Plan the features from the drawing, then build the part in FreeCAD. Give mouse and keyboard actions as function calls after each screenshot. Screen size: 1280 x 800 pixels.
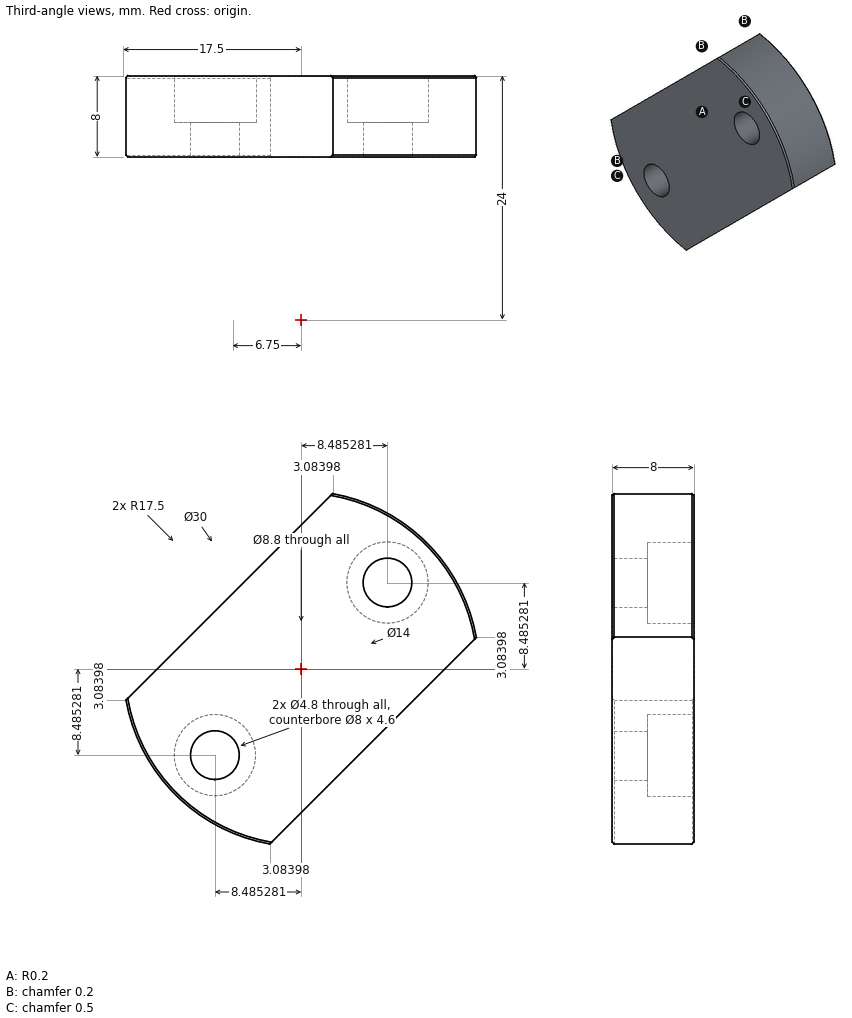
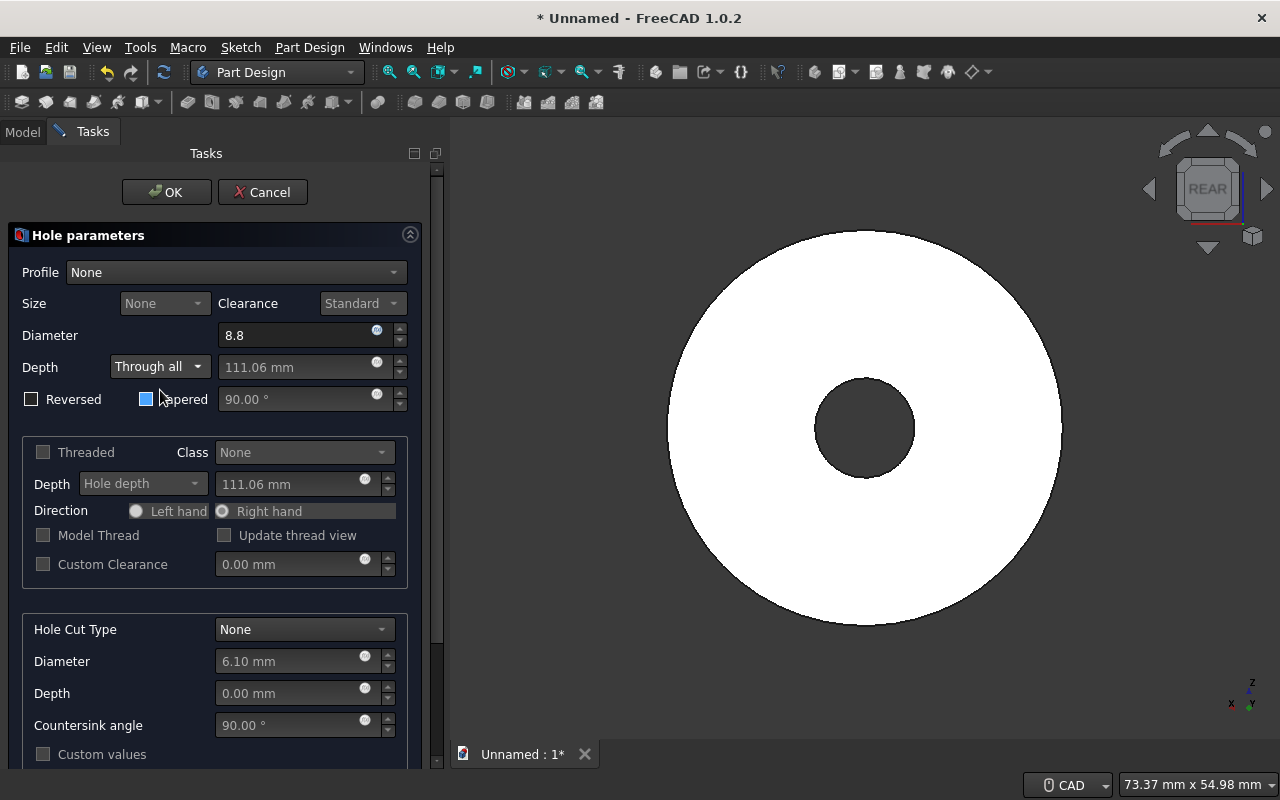
click(167, 192)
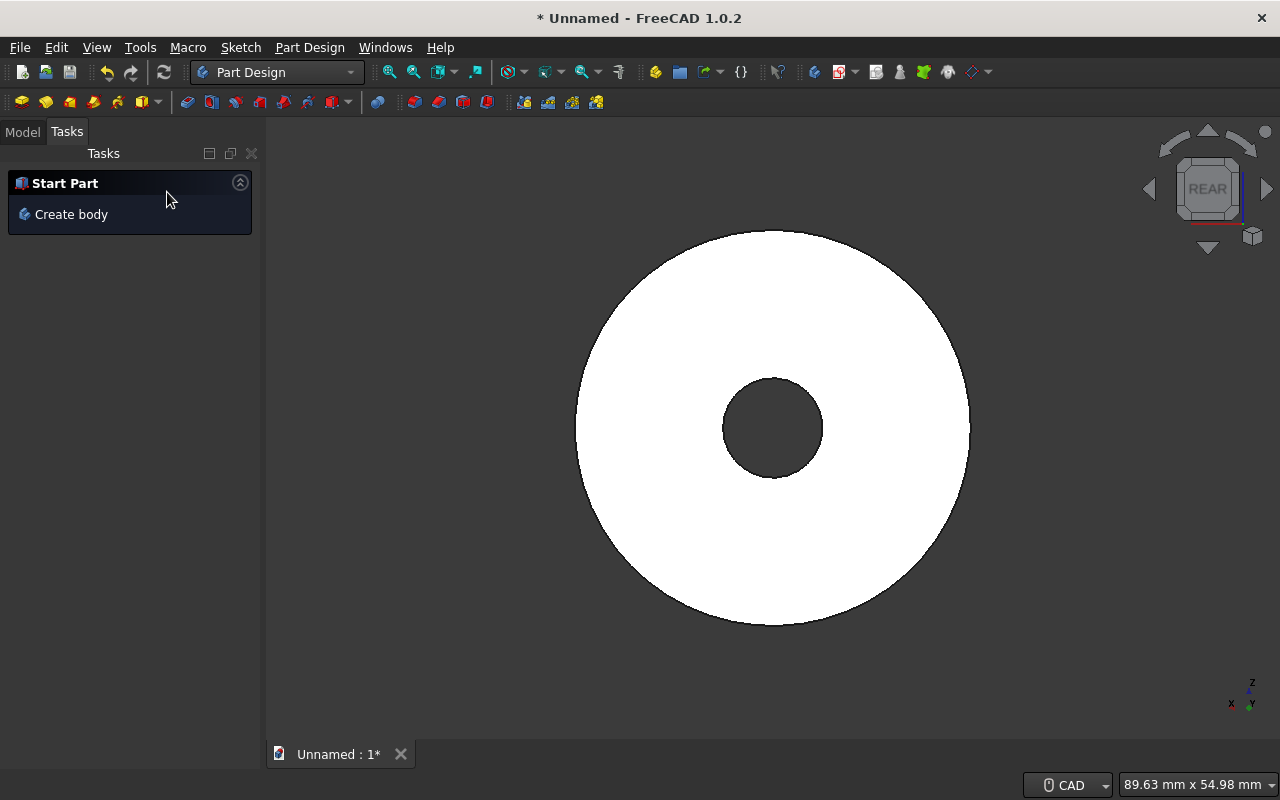
click(660, 370)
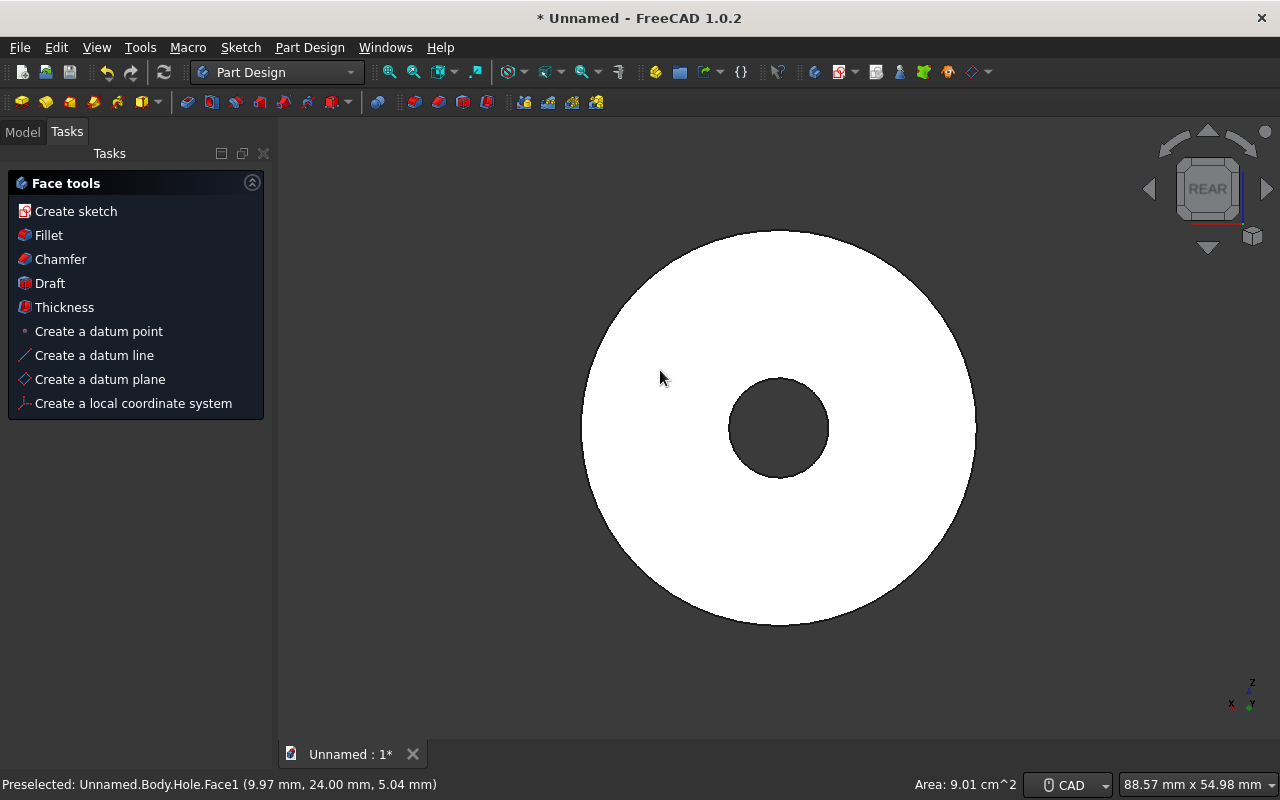
click(840, 72)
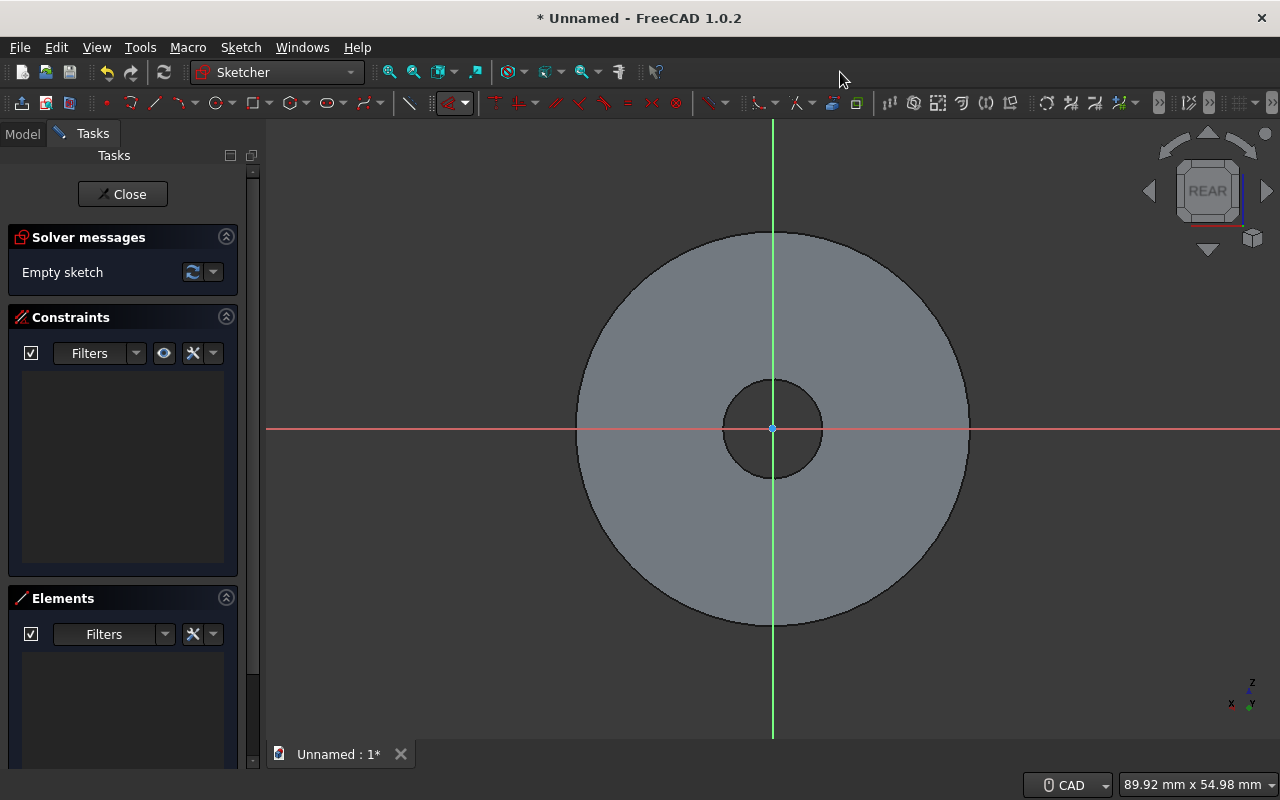
scroll(912, 429, up, 2)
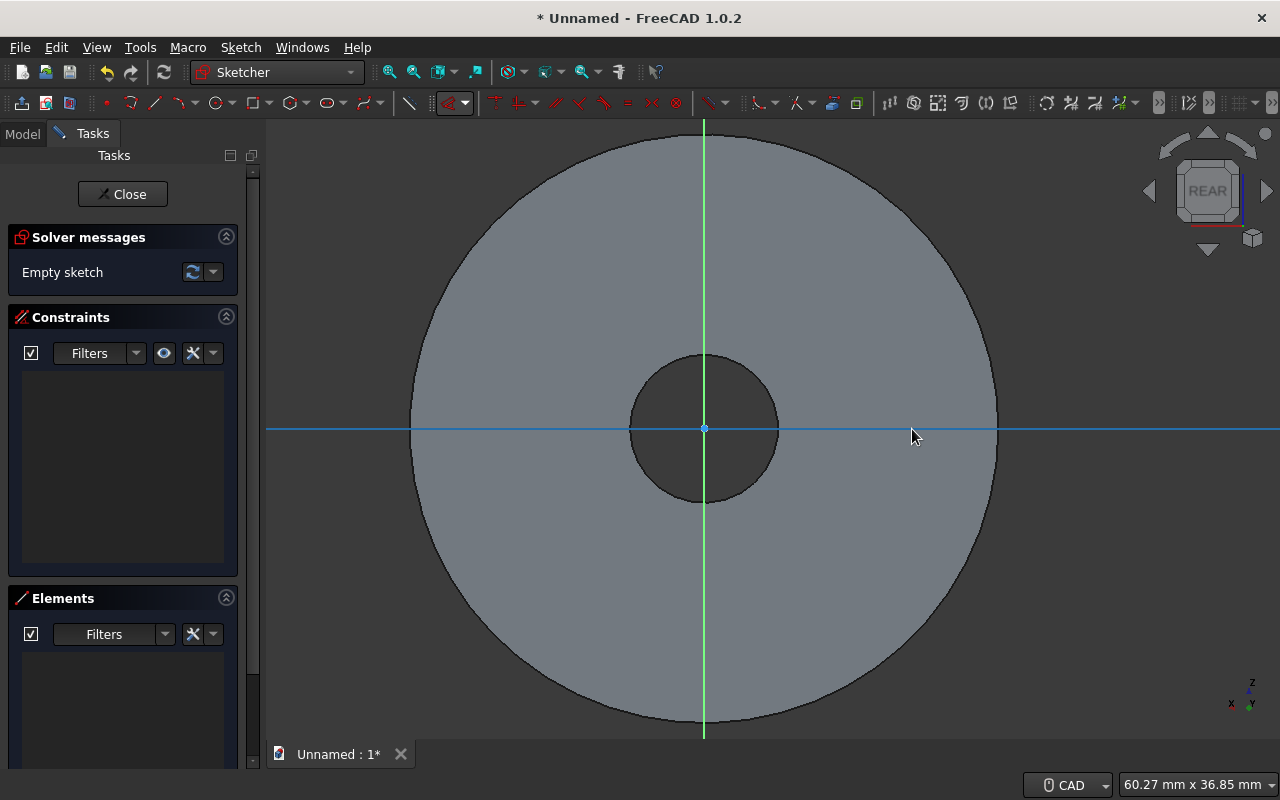
click(216, 104)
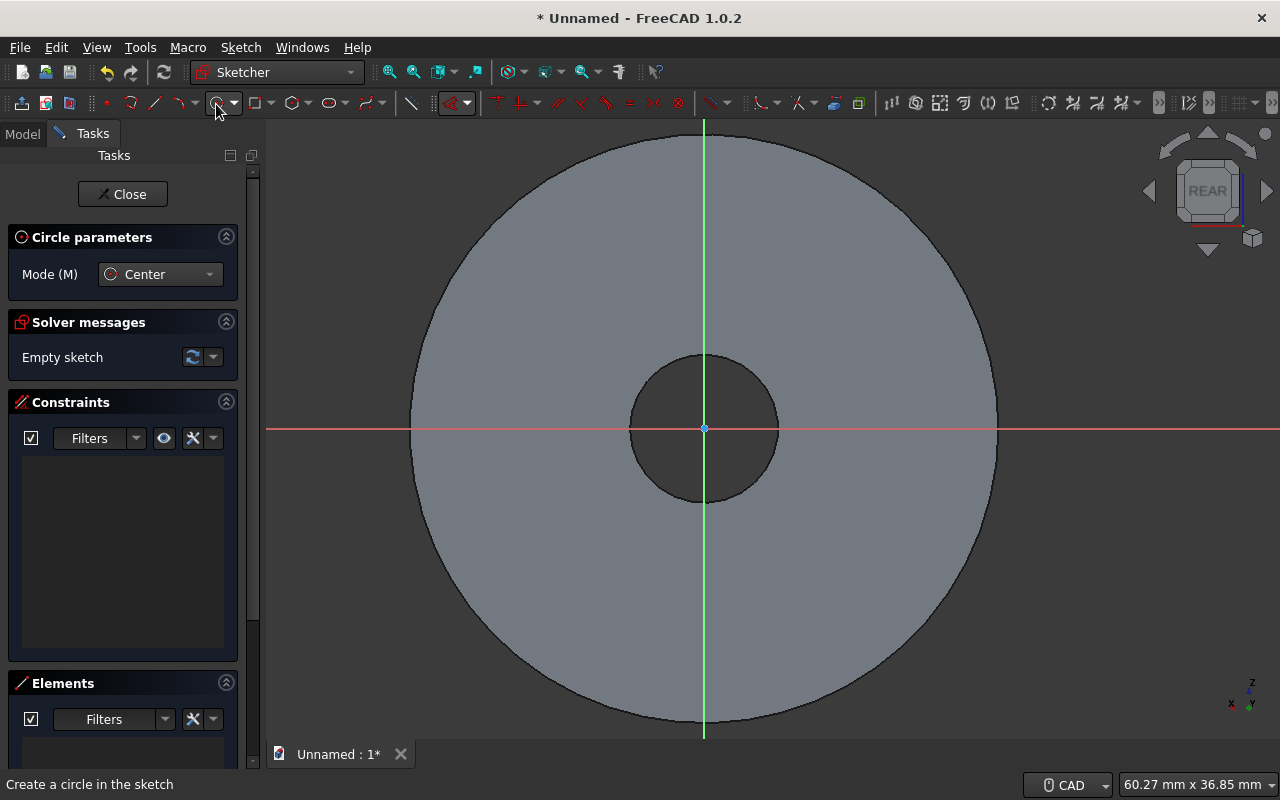
click(847, 572)
move(875, 543)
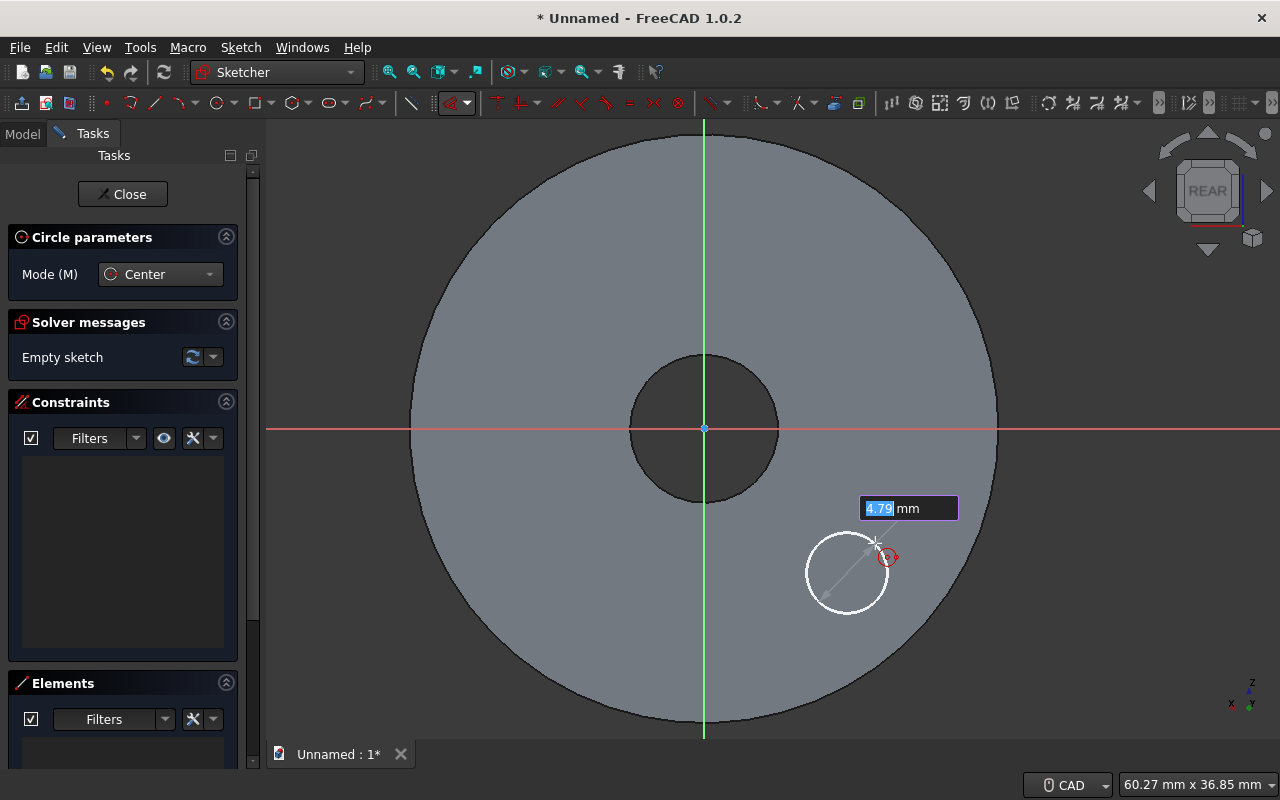
text(4.8)
key(Return)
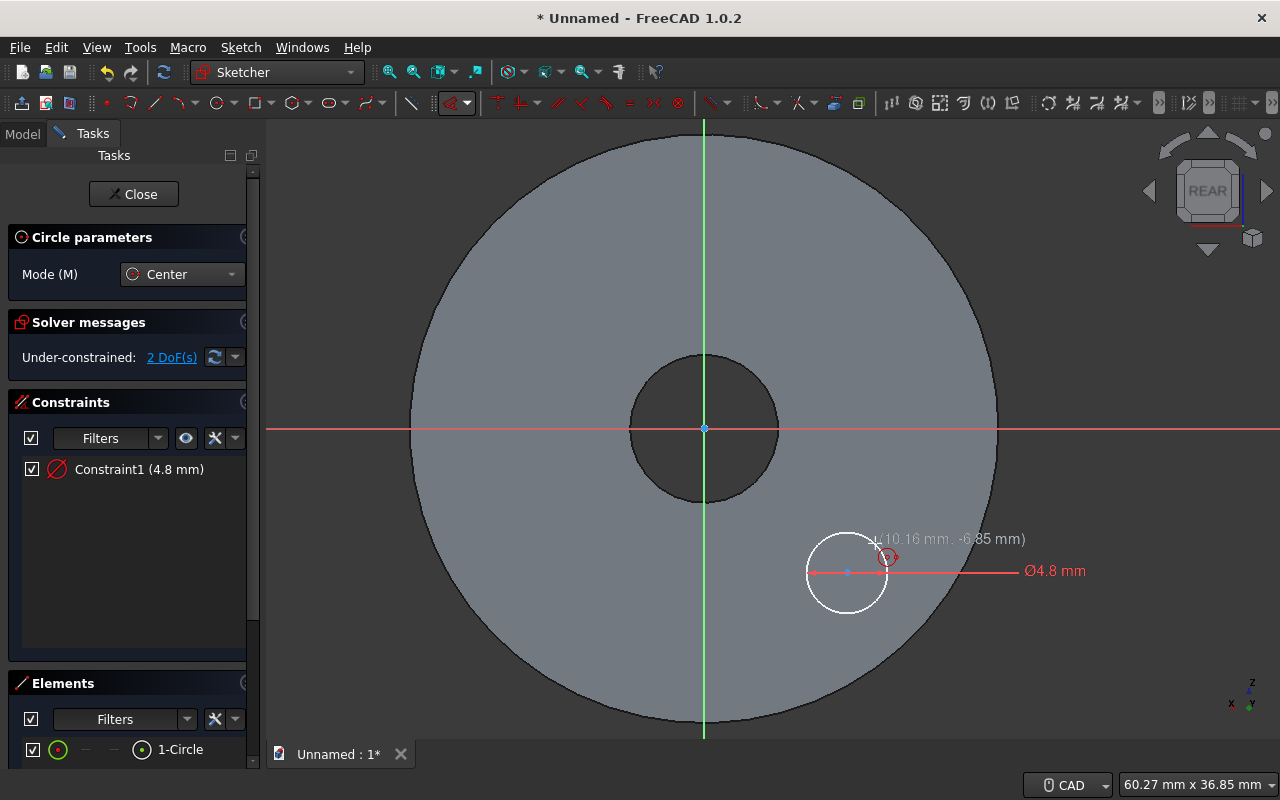
click(561, 286)
move(590, 257)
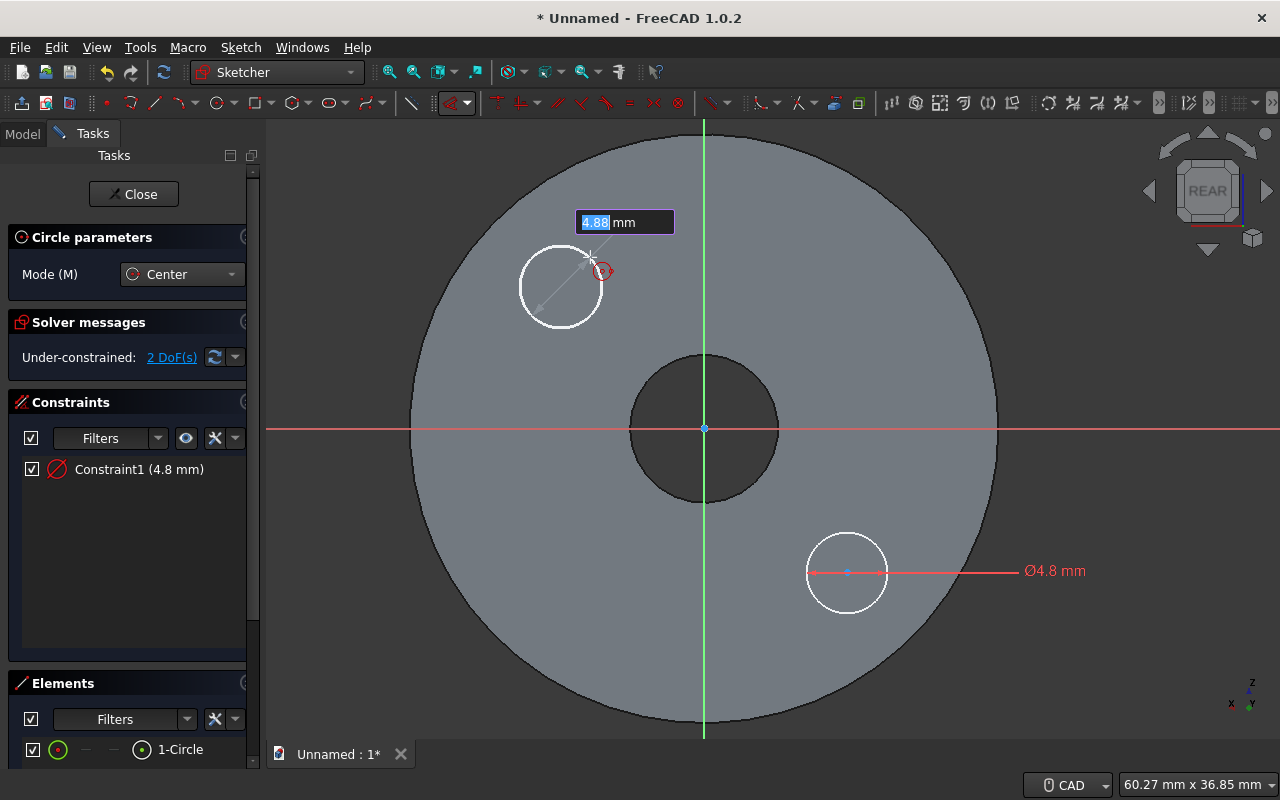
text(4.8)
key(Return)
key(Escape)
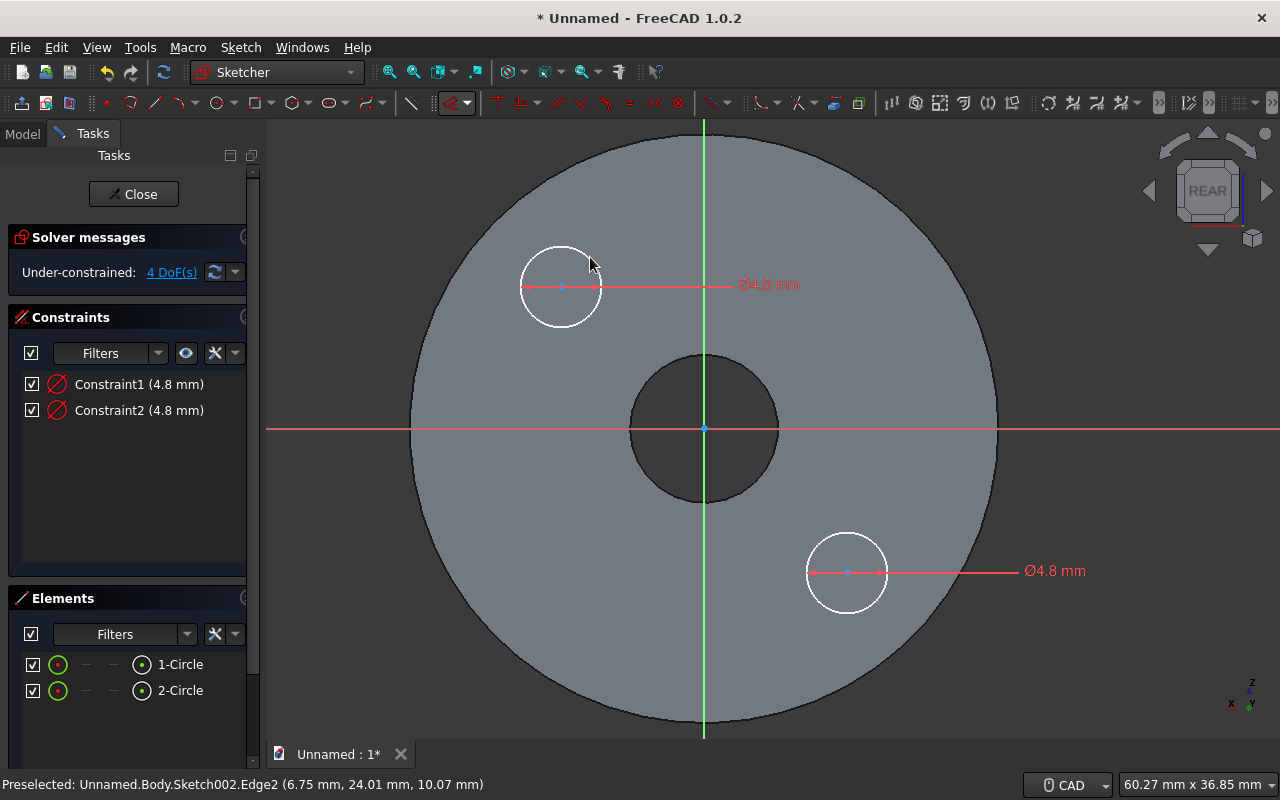
click(847, 573)